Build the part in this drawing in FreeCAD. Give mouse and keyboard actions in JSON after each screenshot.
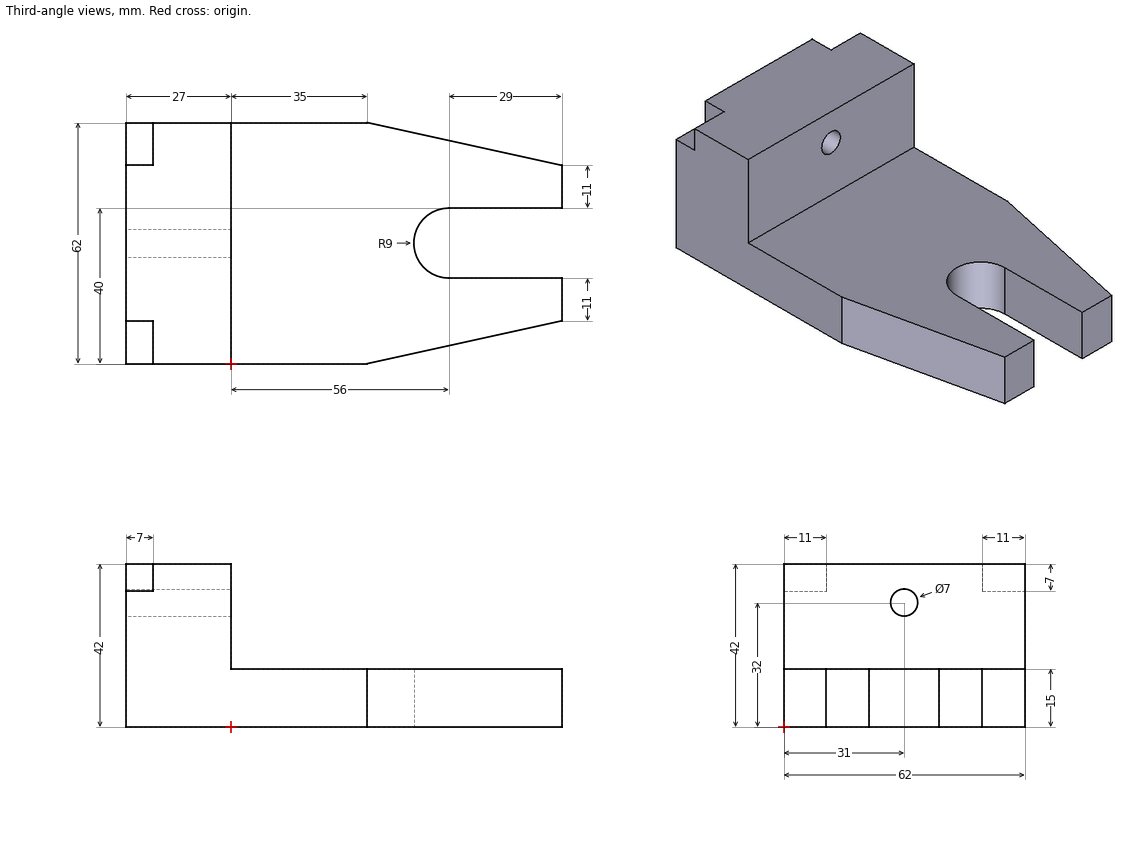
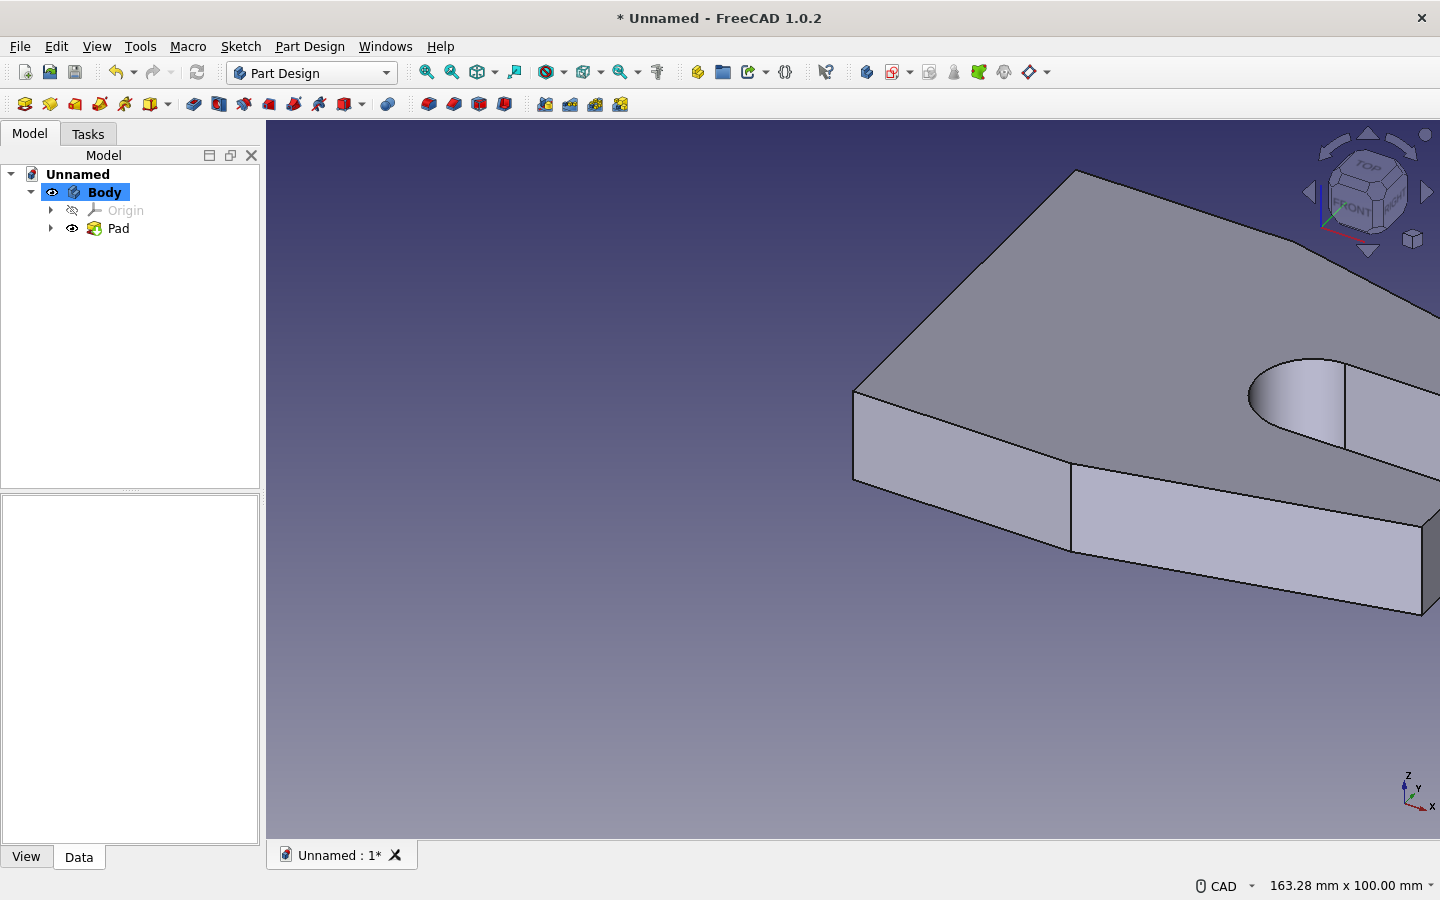
{"action": "left_click", "coordinate": [427, 72]}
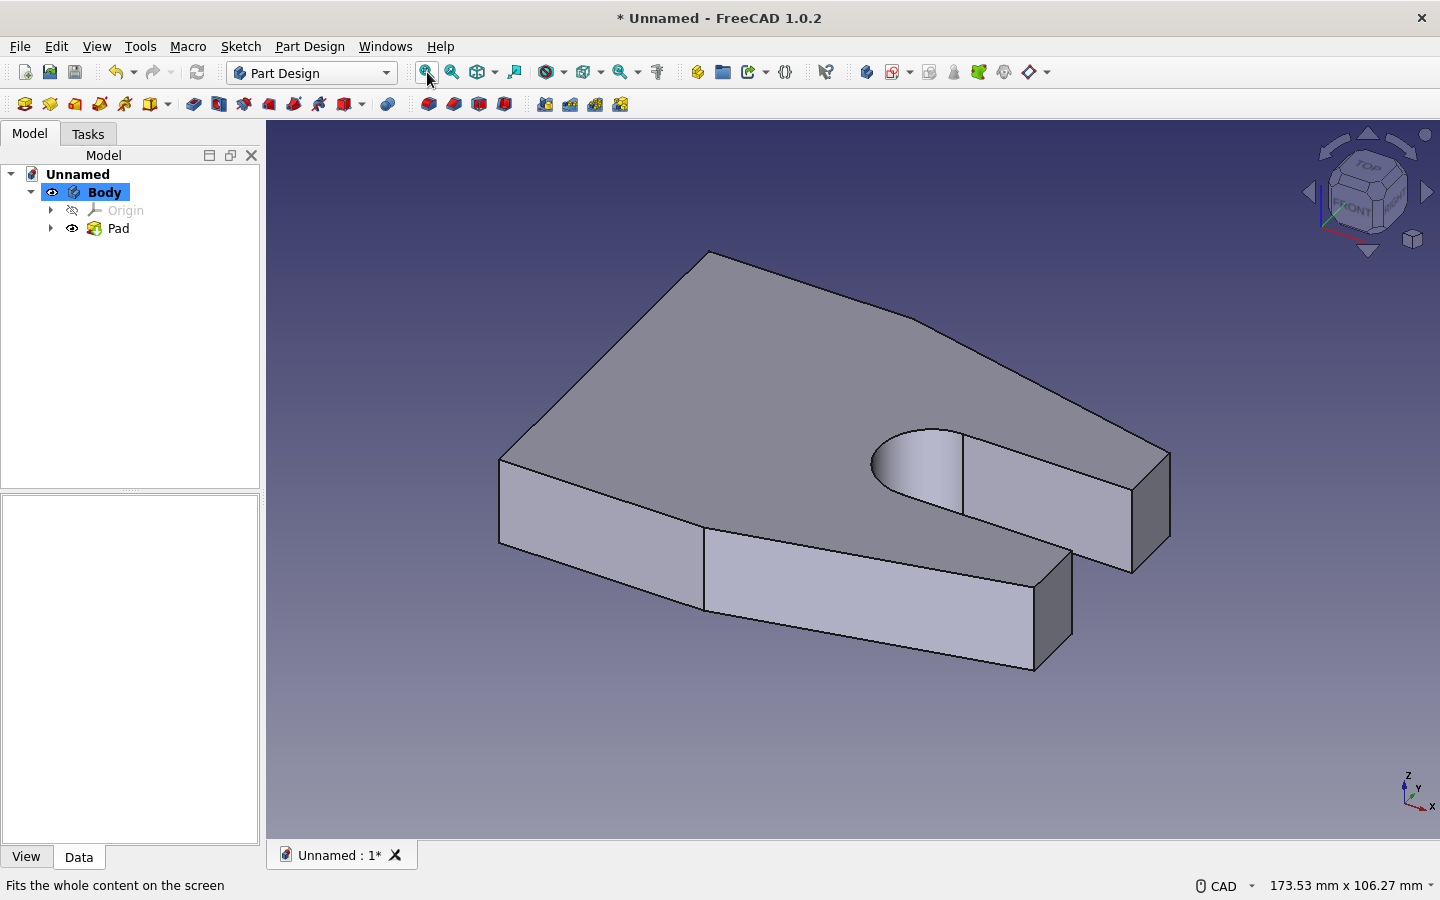
{"action": "left_click", "coordinate": [892, 72]}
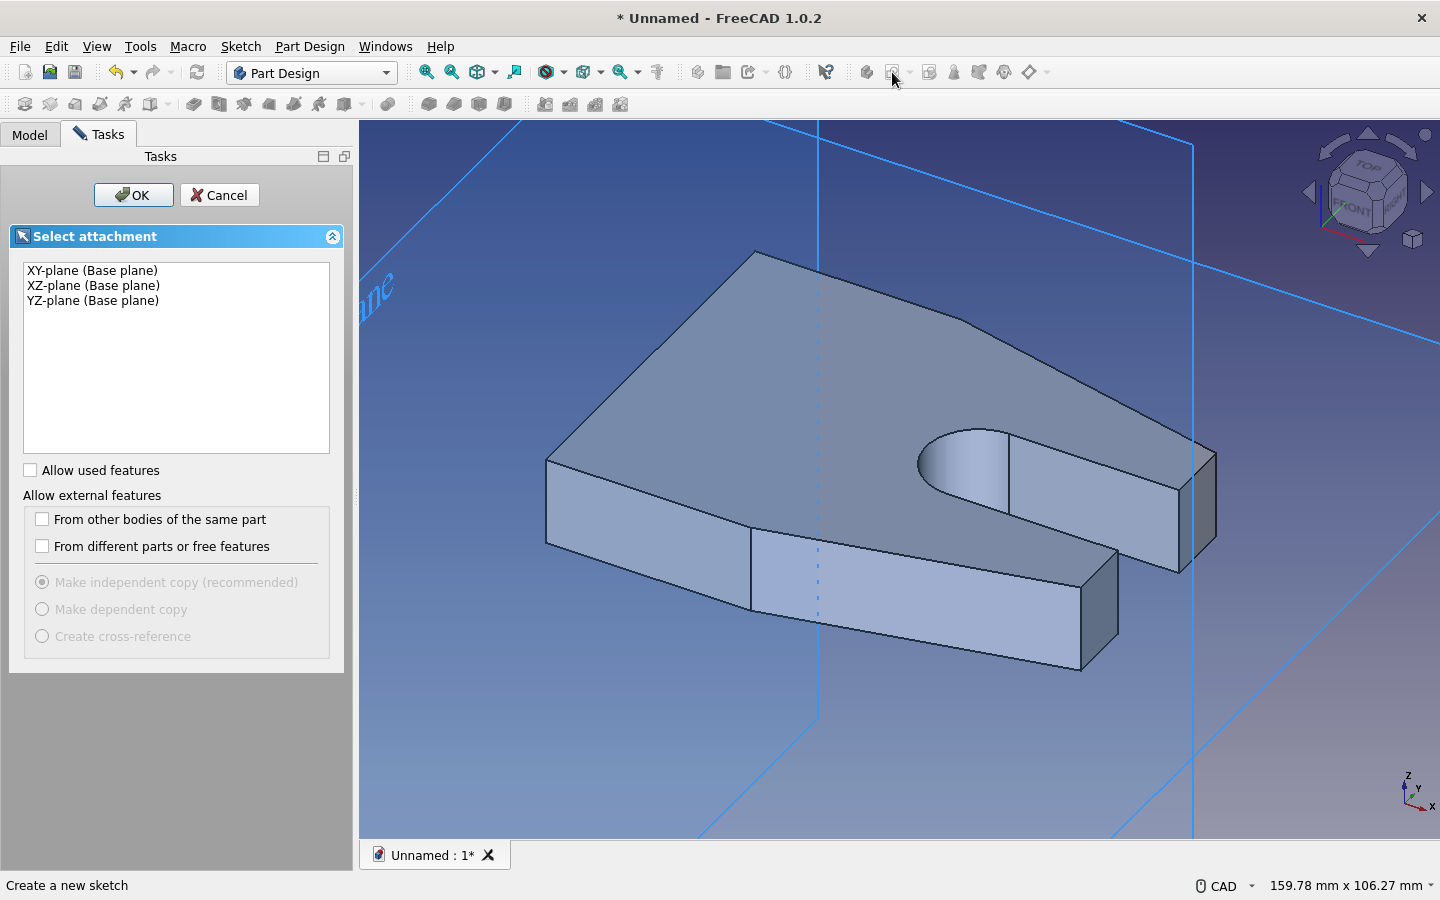
{"action": "left_click", "coordinate": [84, 270]}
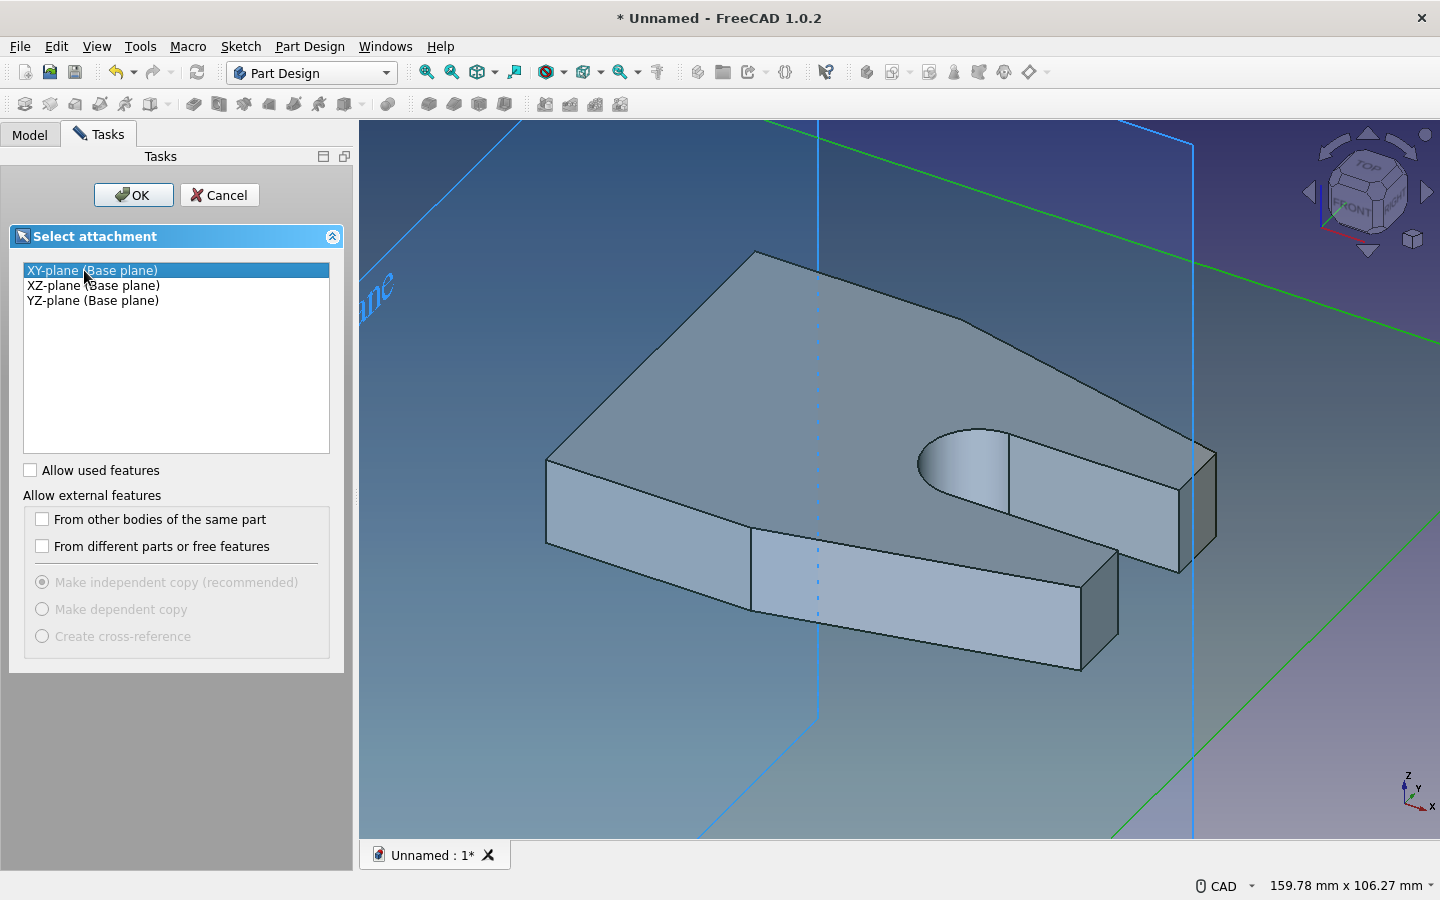
{"action": "left_click", "coordinate": [134, 195]}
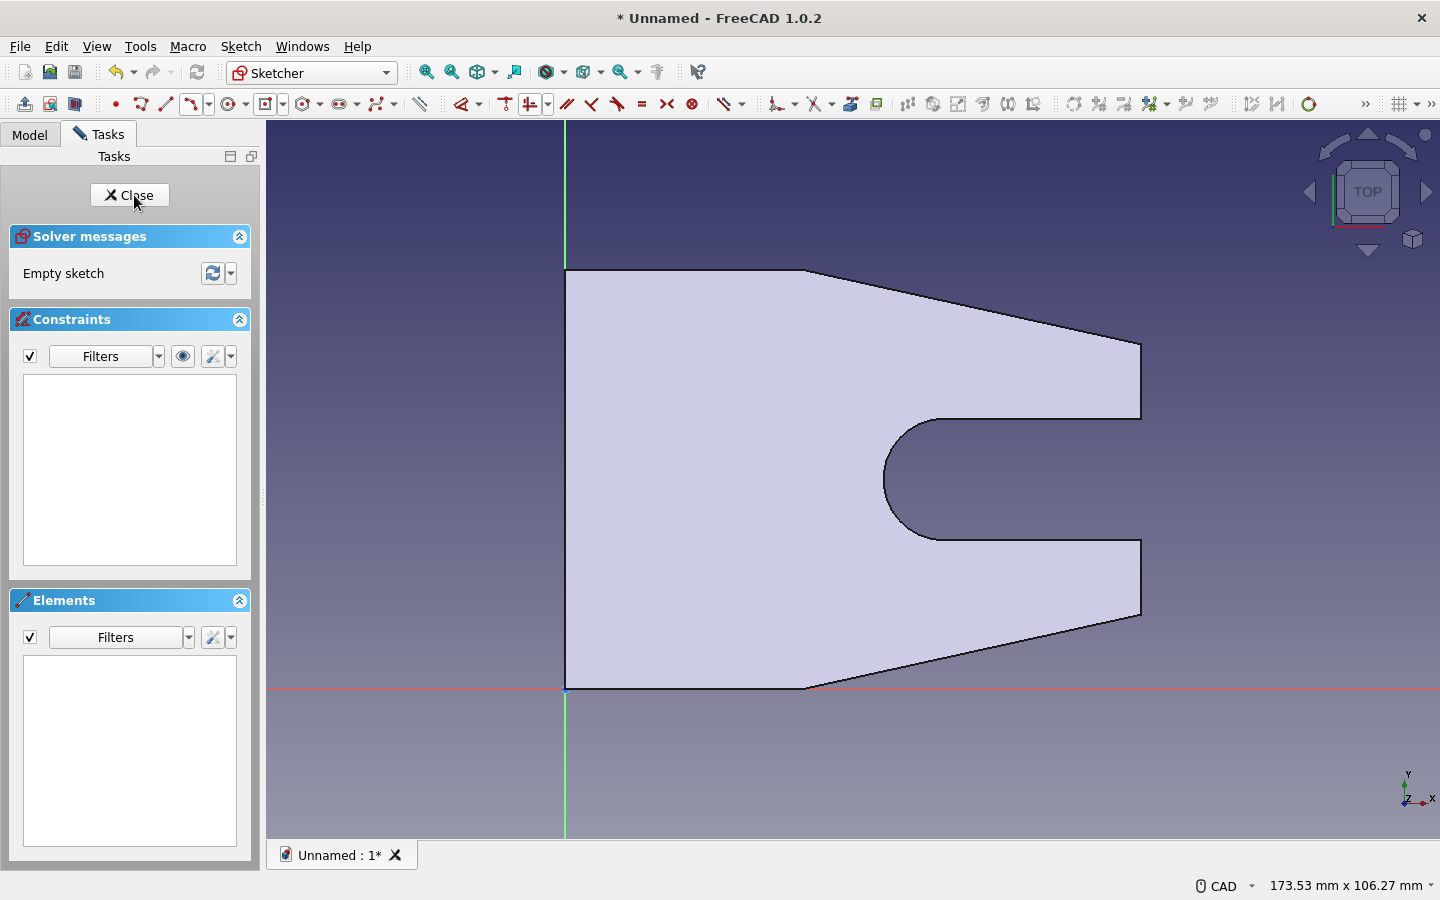
{"action": "left_click", "coordinate": [75, 104]}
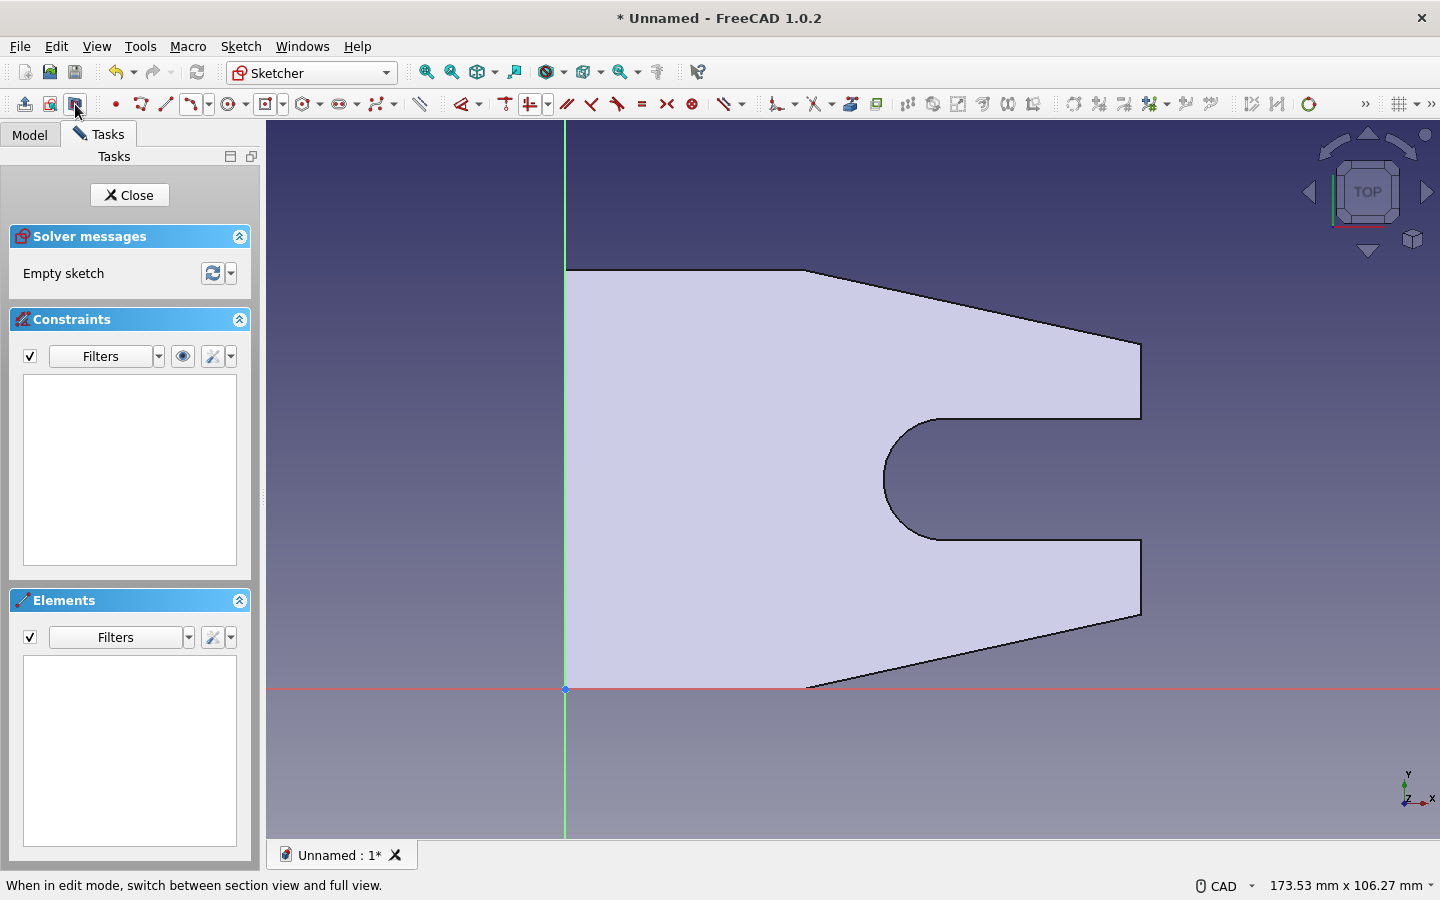
{"action": "key", "text": "g r"}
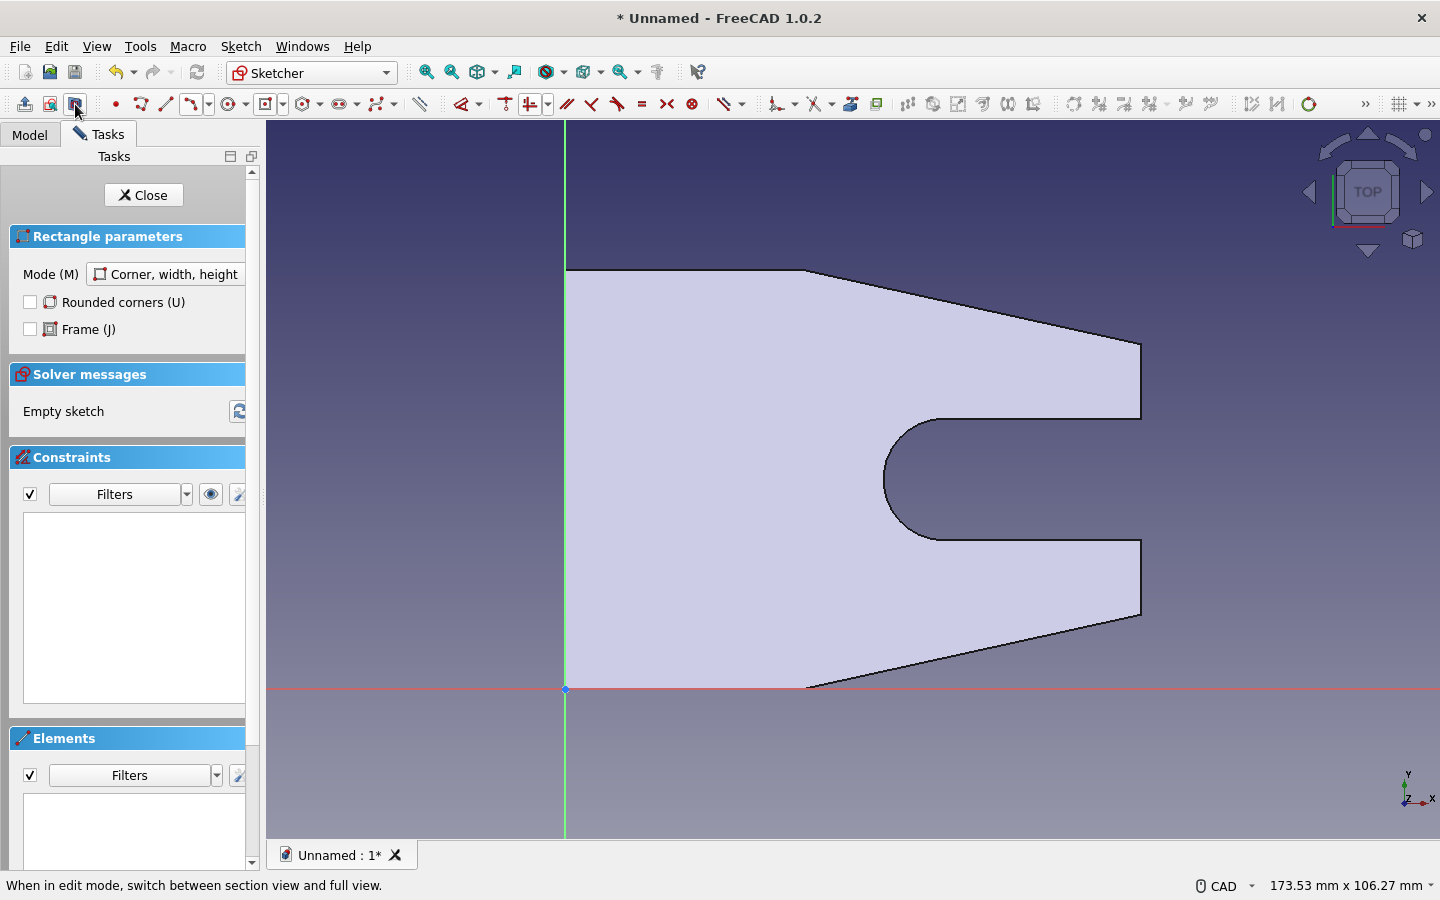
{"action": "left_click", "coordinate": [565, 689]}
{"action": "left_click", "coordinate": [383, 270]}
{"action": "key", "text": "Escape"}